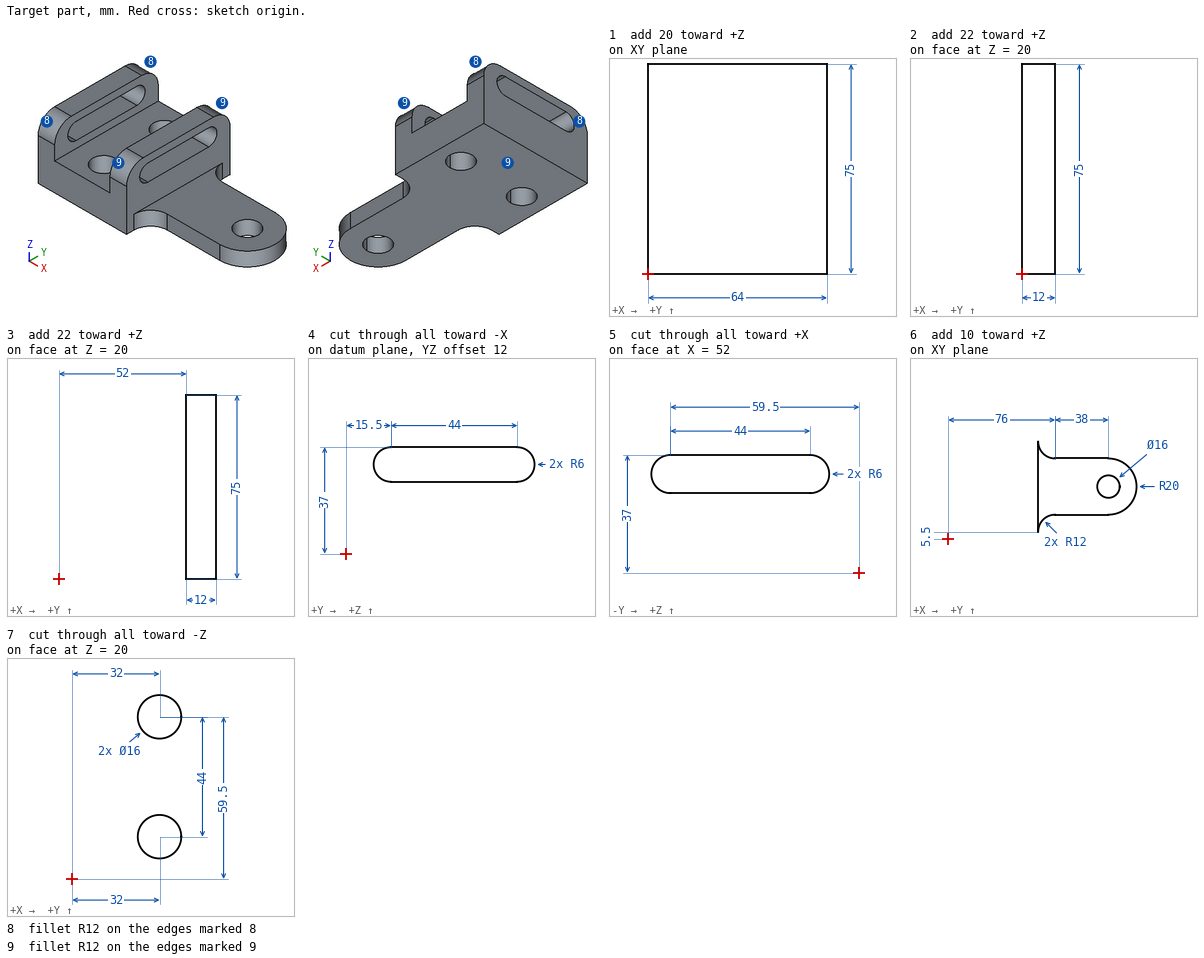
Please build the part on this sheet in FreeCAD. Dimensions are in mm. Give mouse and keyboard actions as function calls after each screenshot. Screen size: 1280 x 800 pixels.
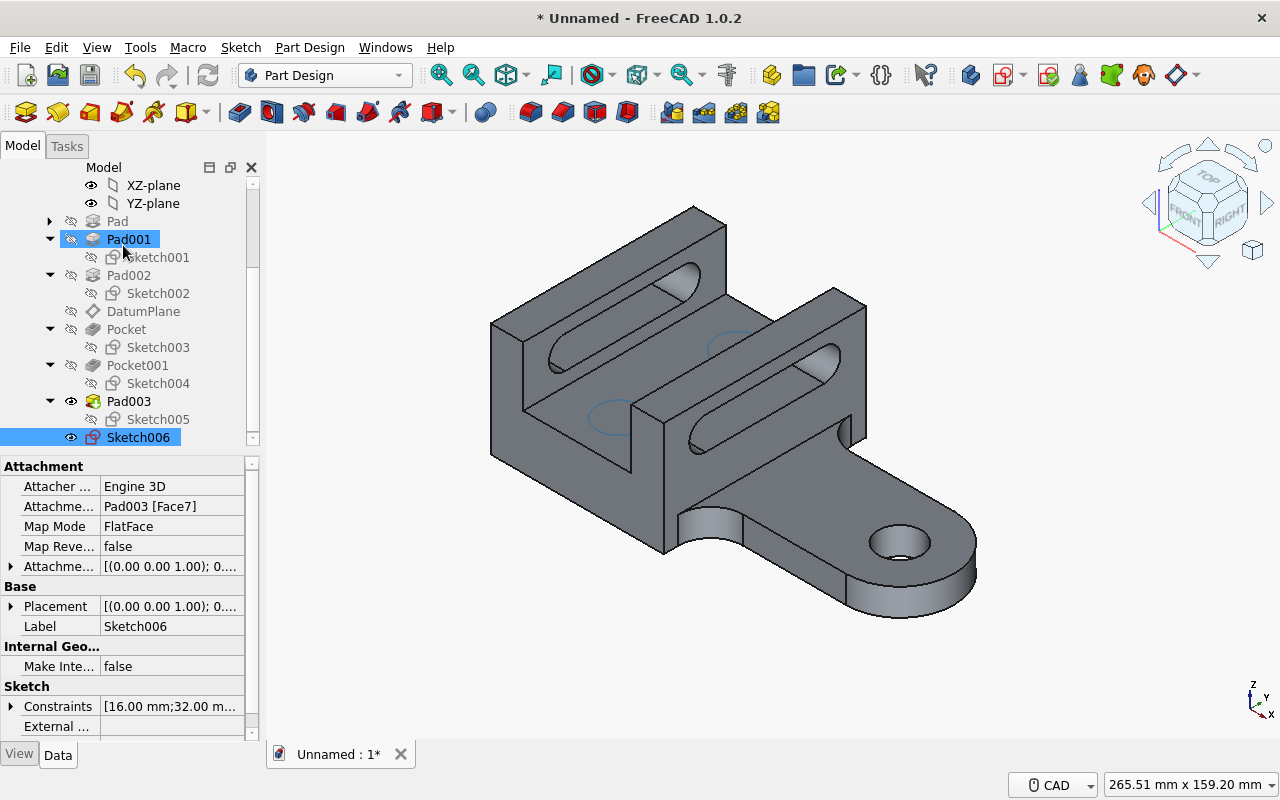
click(240, 112)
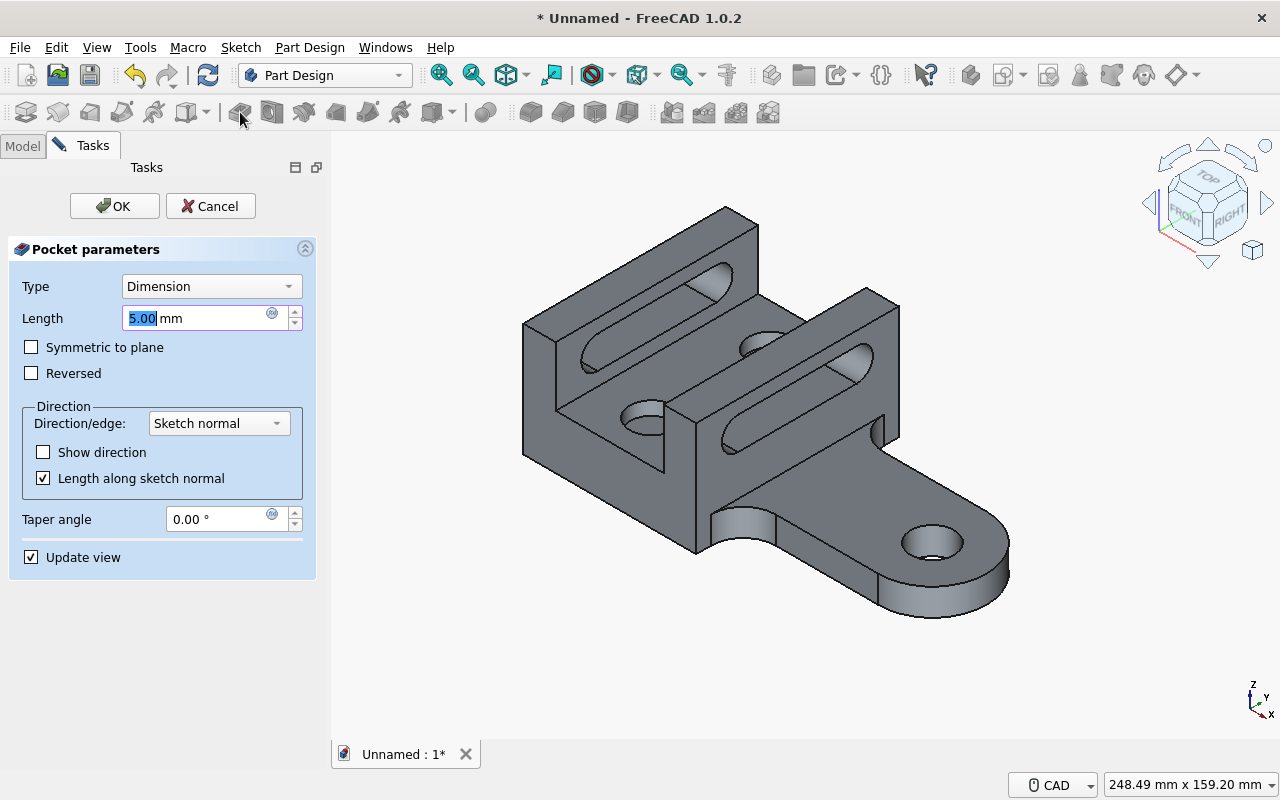
click(212, 286)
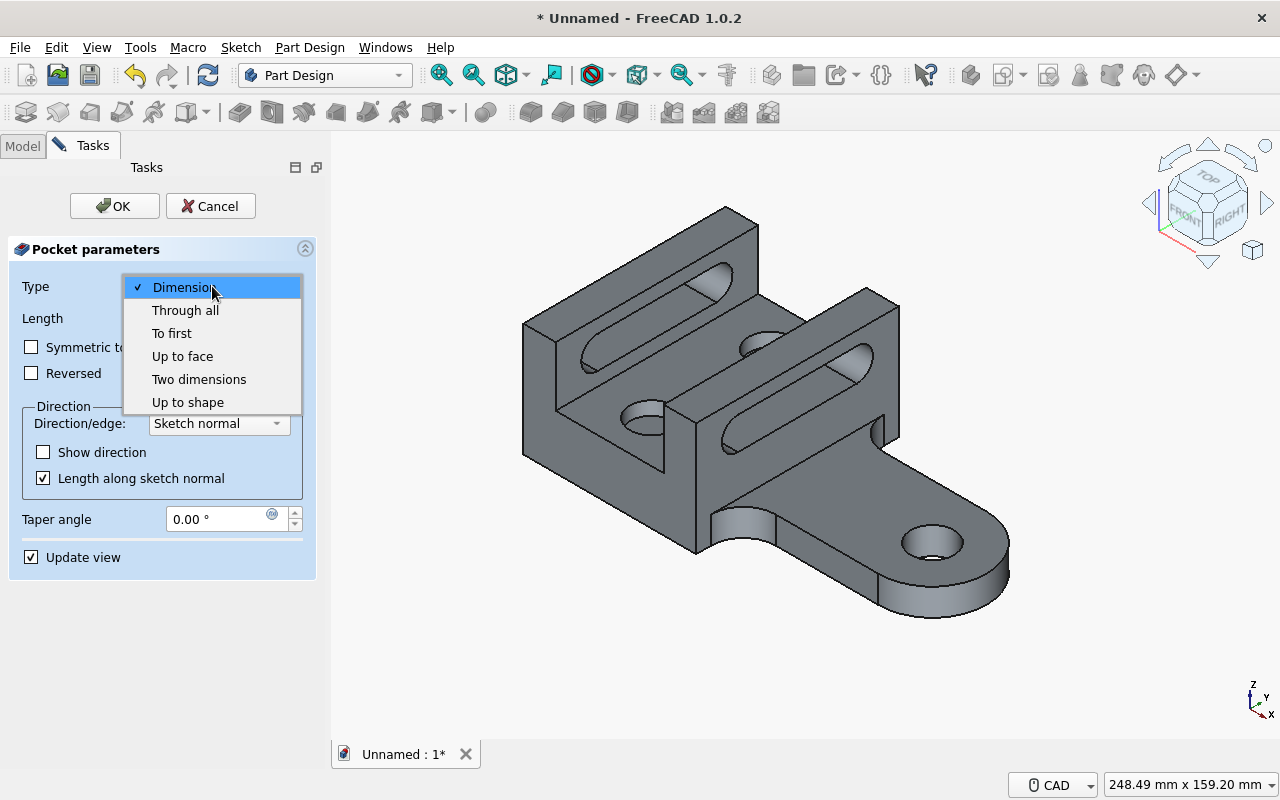
click(212, 310)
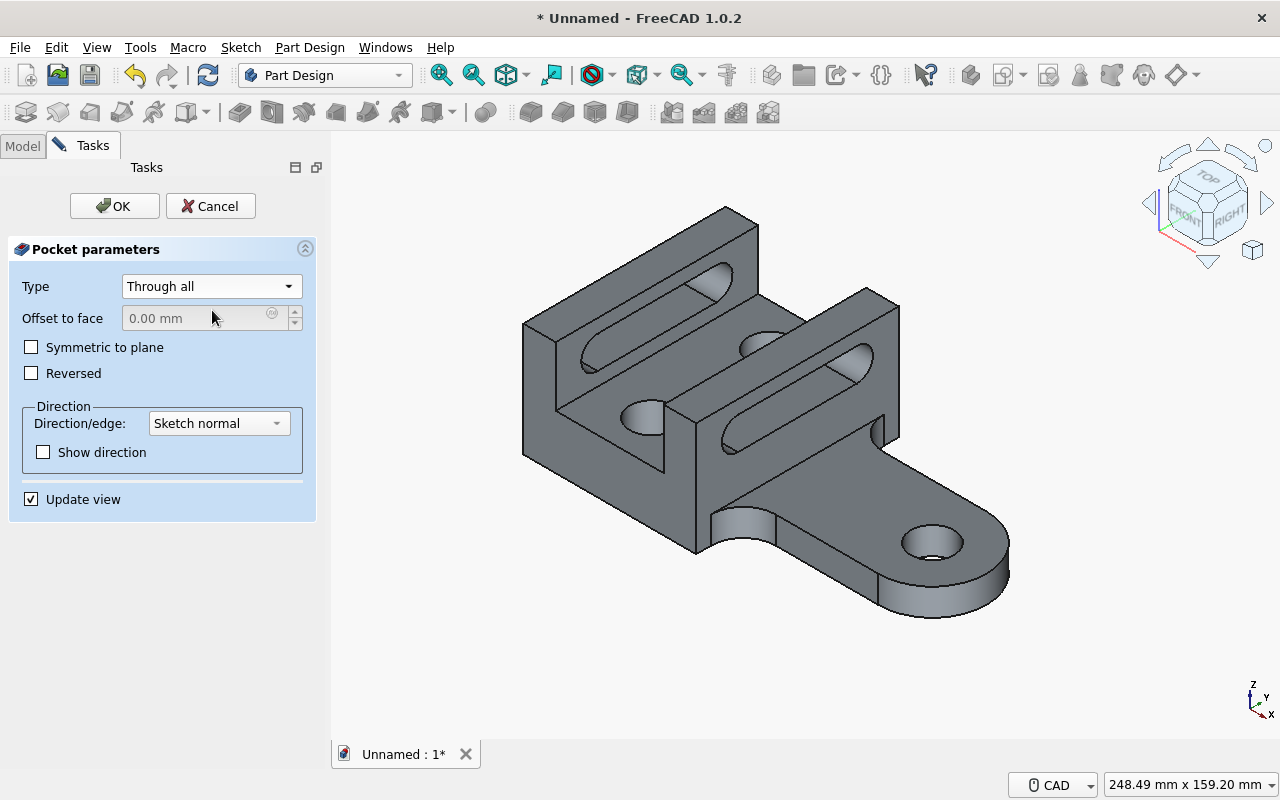
click(115, 206)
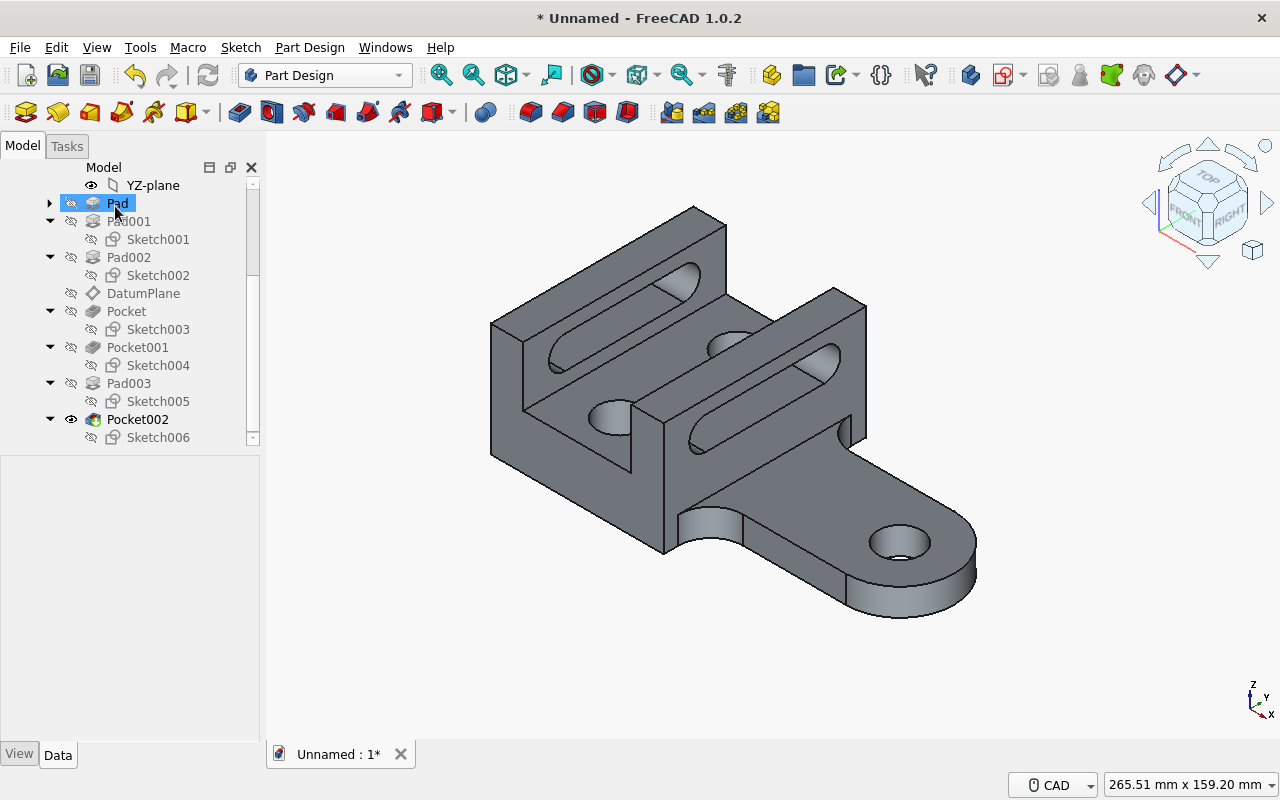
click(507, 332)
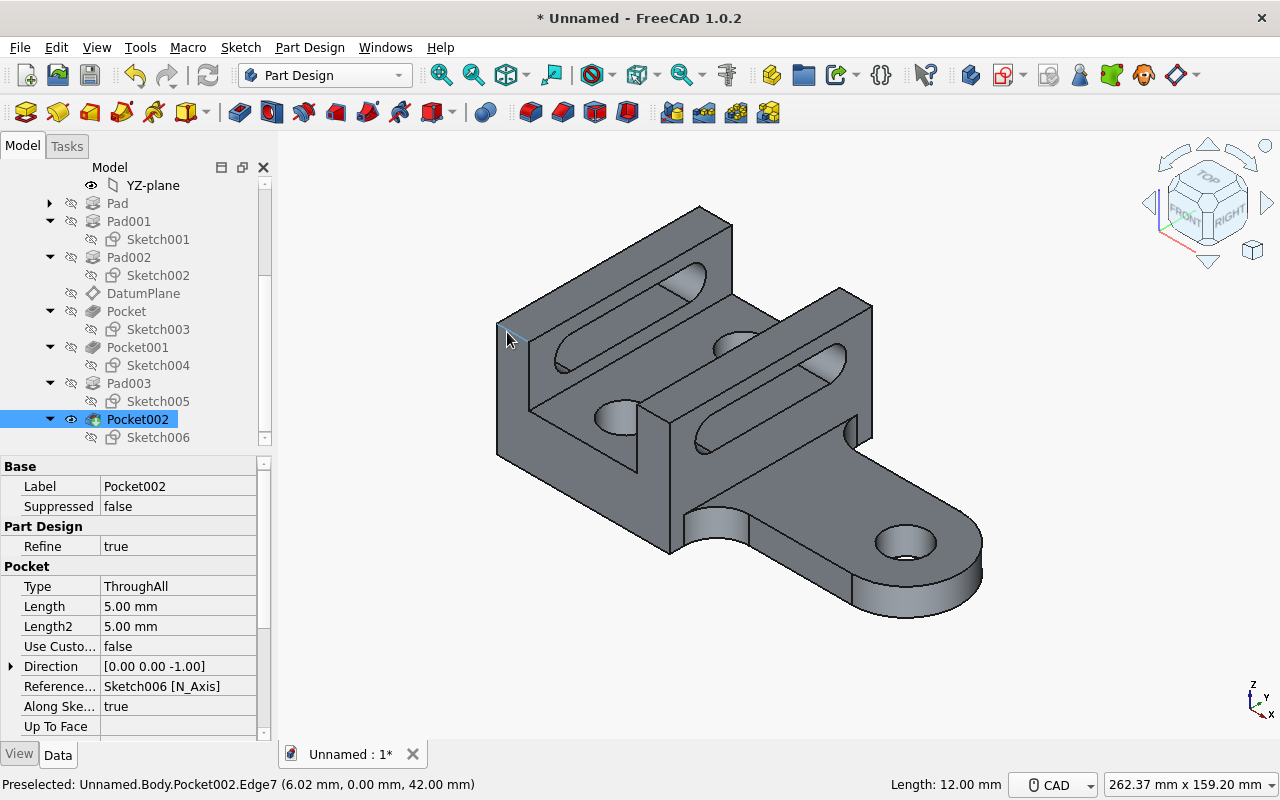
key(2)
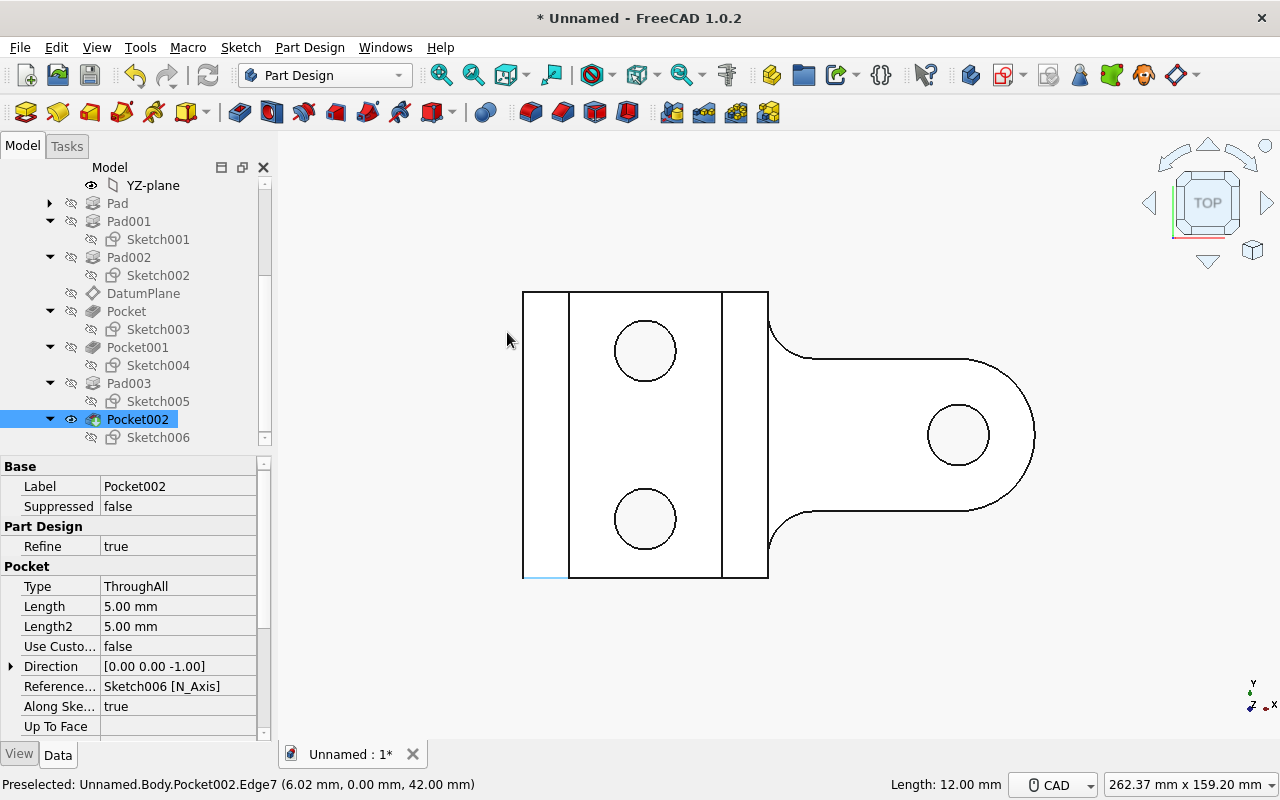
click(546, 291, ctrl)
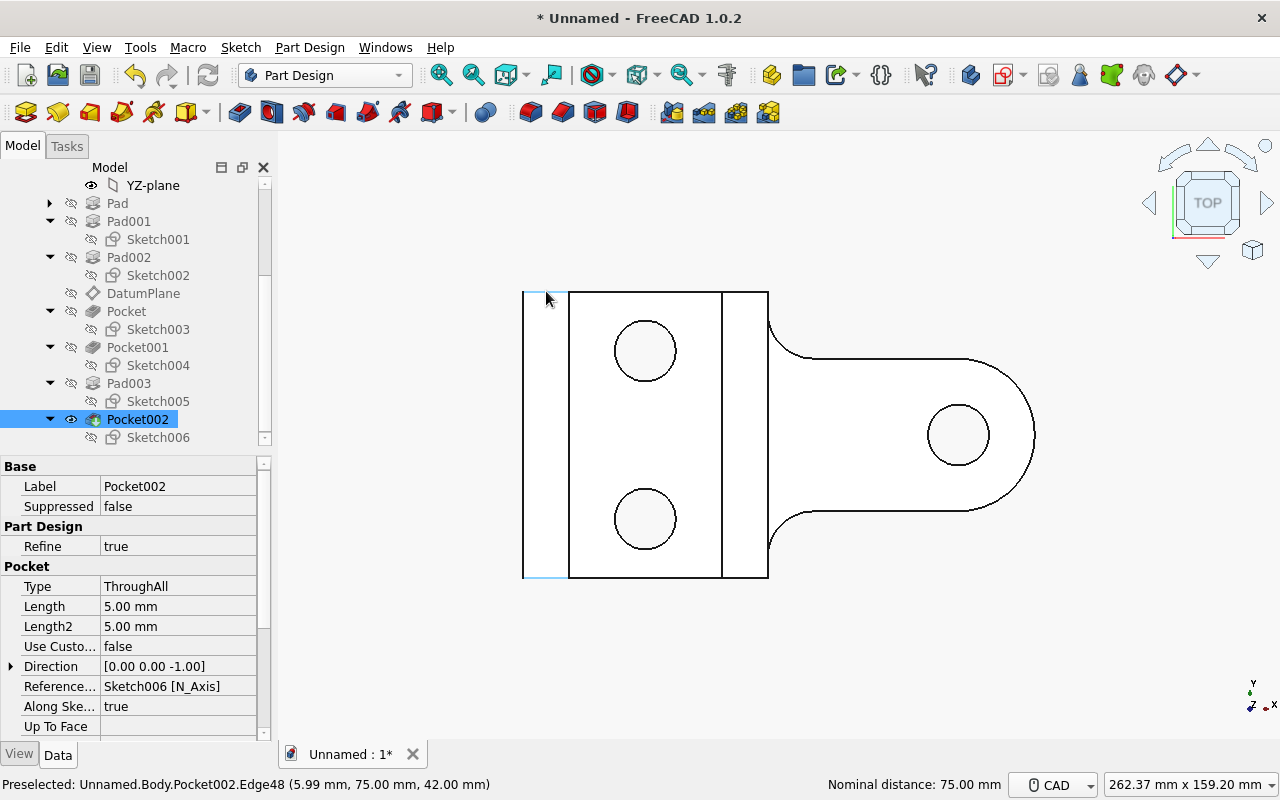
click(532, 112)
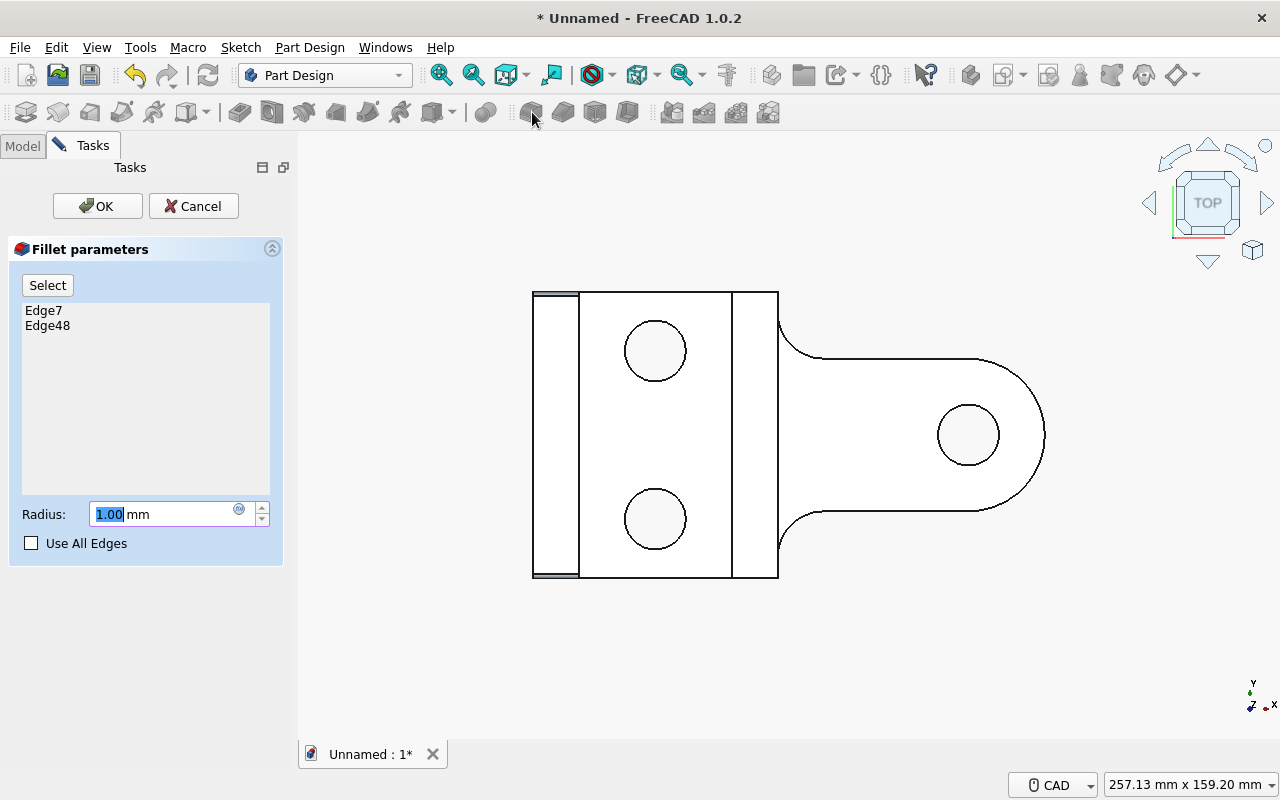
text(12)
key(Tab)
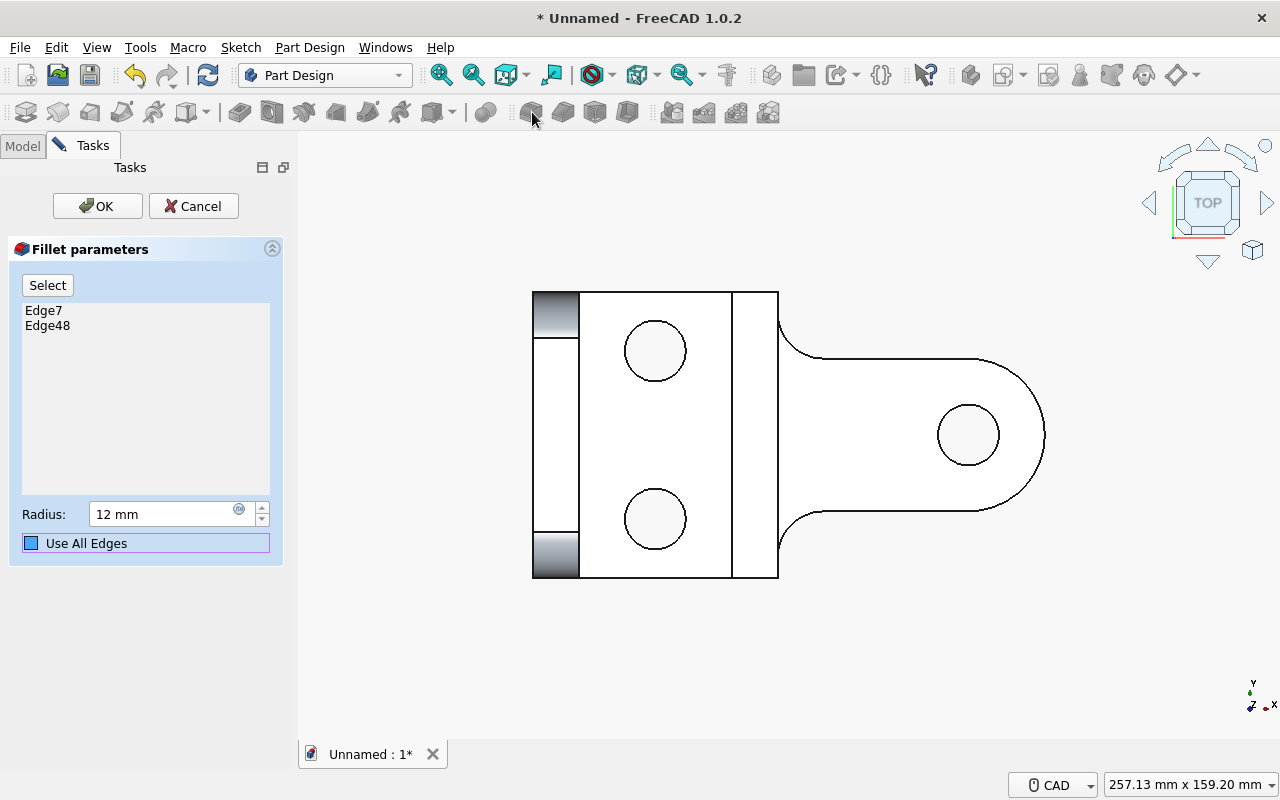
click(98, 206)